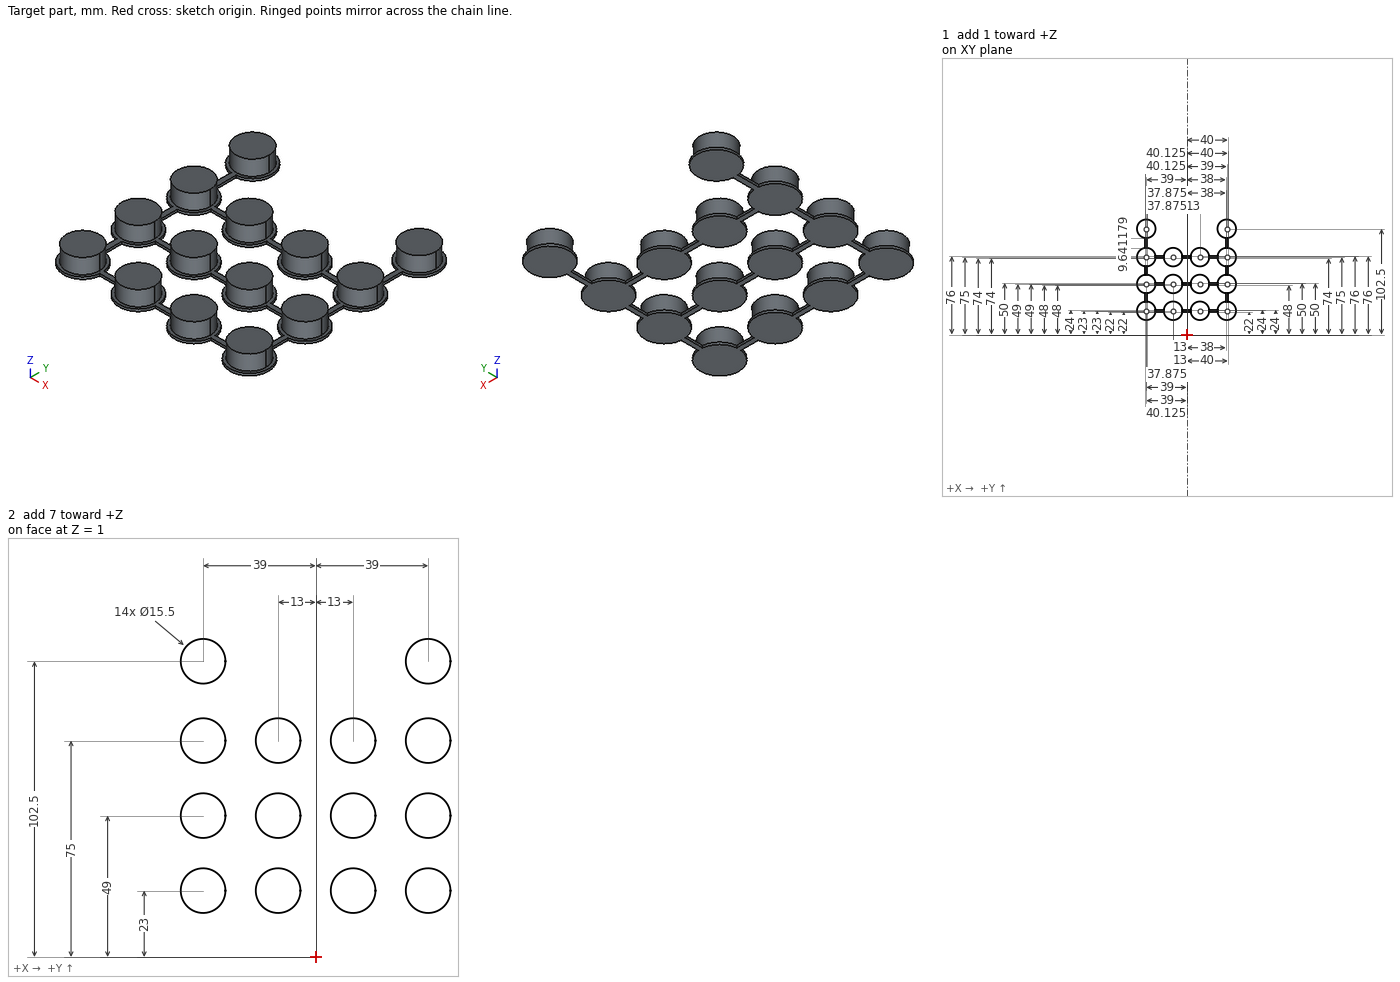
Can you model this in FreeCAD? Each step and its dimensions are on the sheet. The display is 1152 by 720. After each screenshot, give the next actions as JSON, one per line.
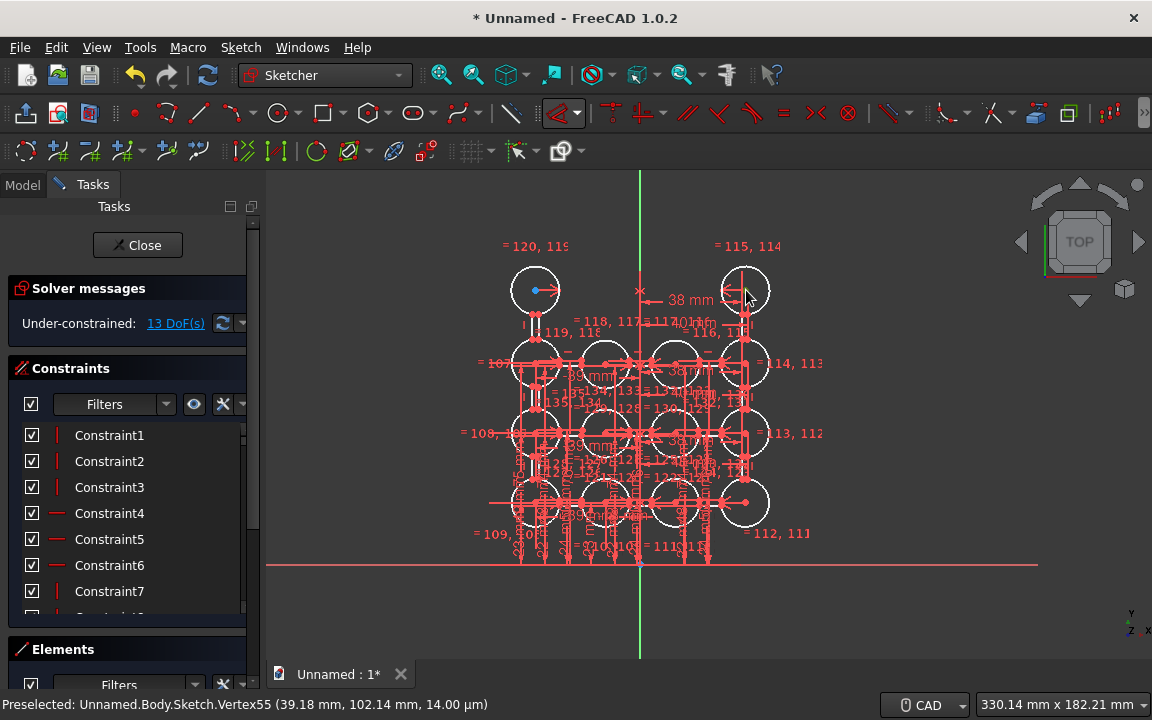
{"action": "key", "text": "l"}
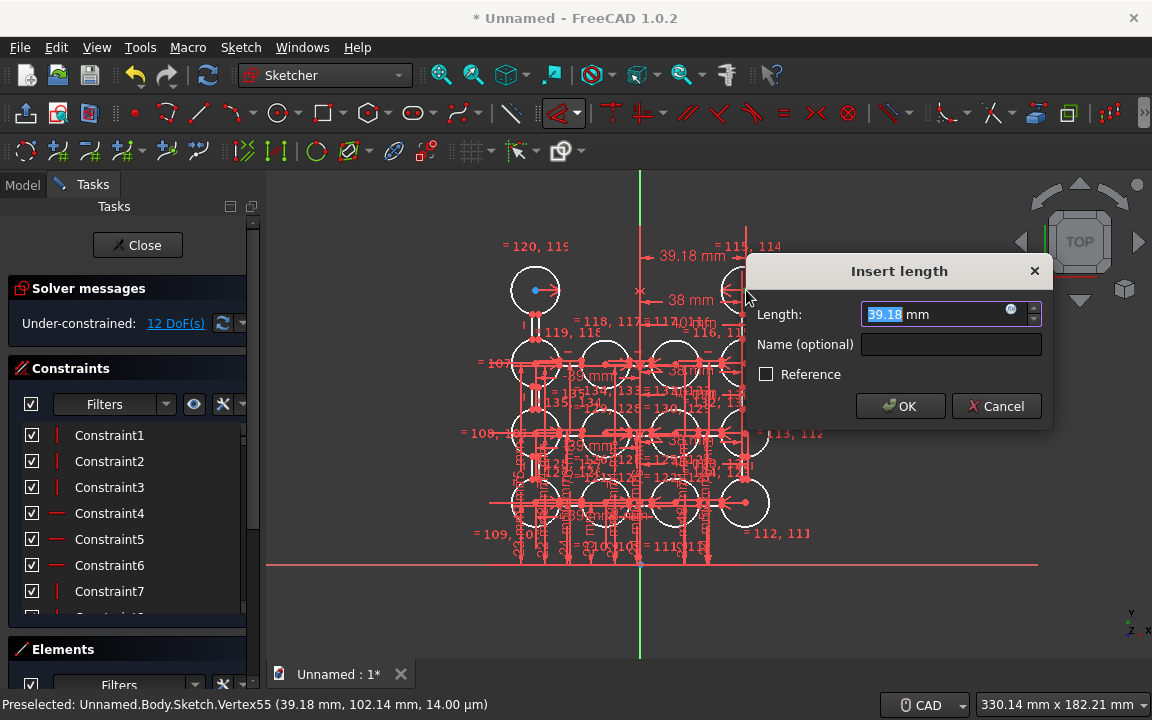
{"action": "type", "text": "39"}
{"action": "key", "text": "Return"}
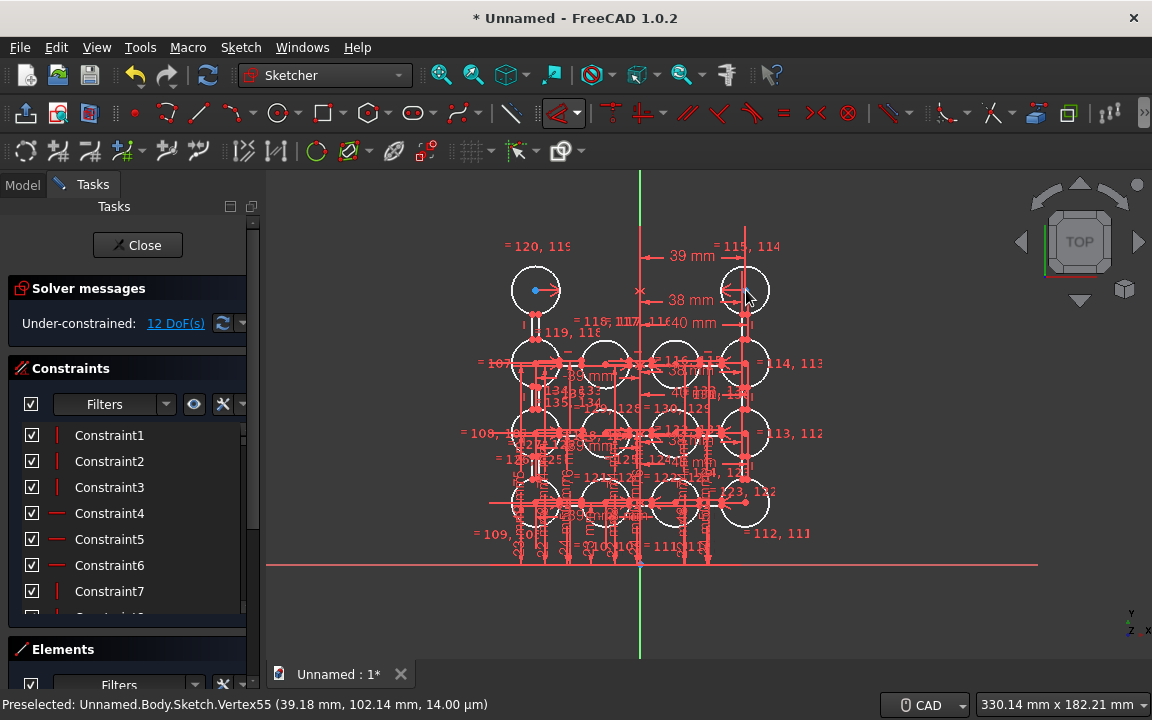
{"action": "left_click", "coordinate": [675, 365]}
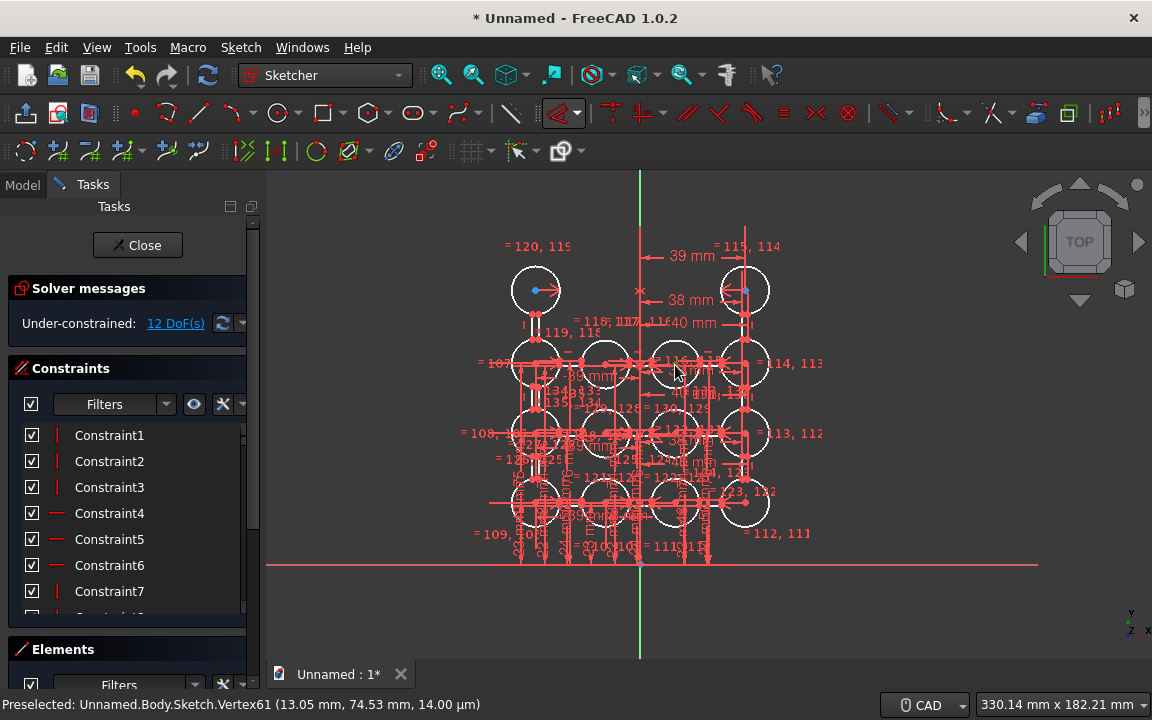
{"action": "left_click", "coordinate": [580, 114]}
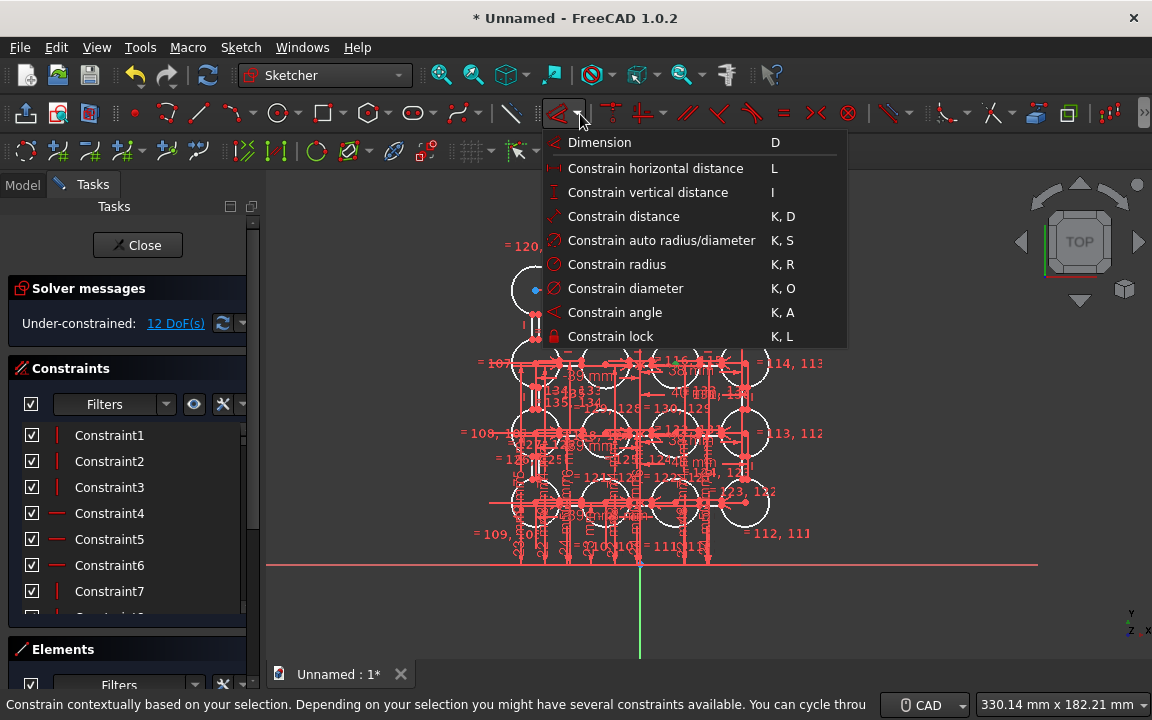
{"action": "left_click", "coordinate": [695, 168]}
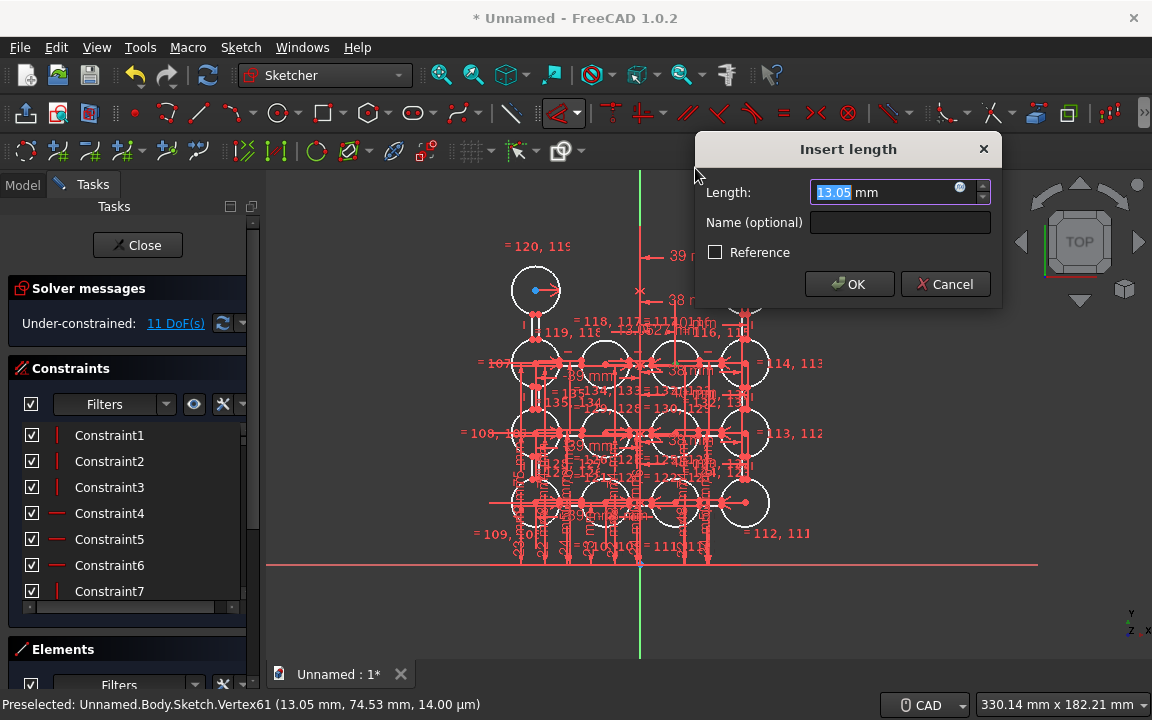
{"action": "type", "text": "13"}
{"action": "key", "text": "Return"}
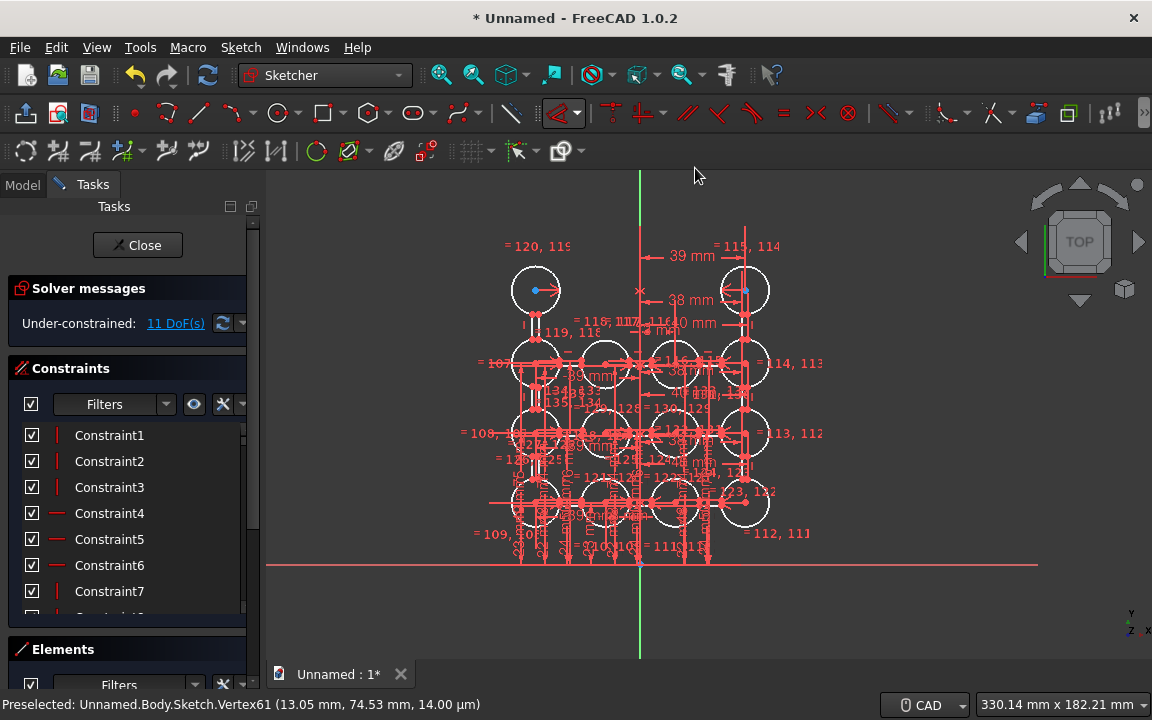
{"action": "left_click", "coordinate": [675, 365]}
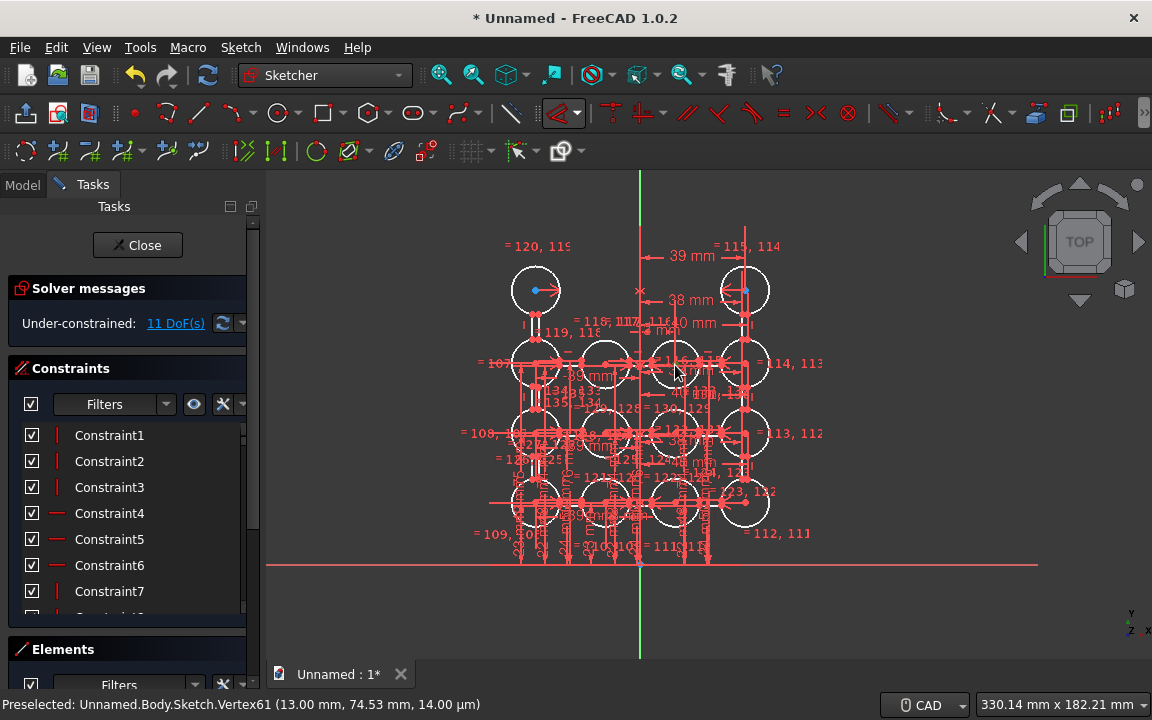
{"action": "key", "text": "i"}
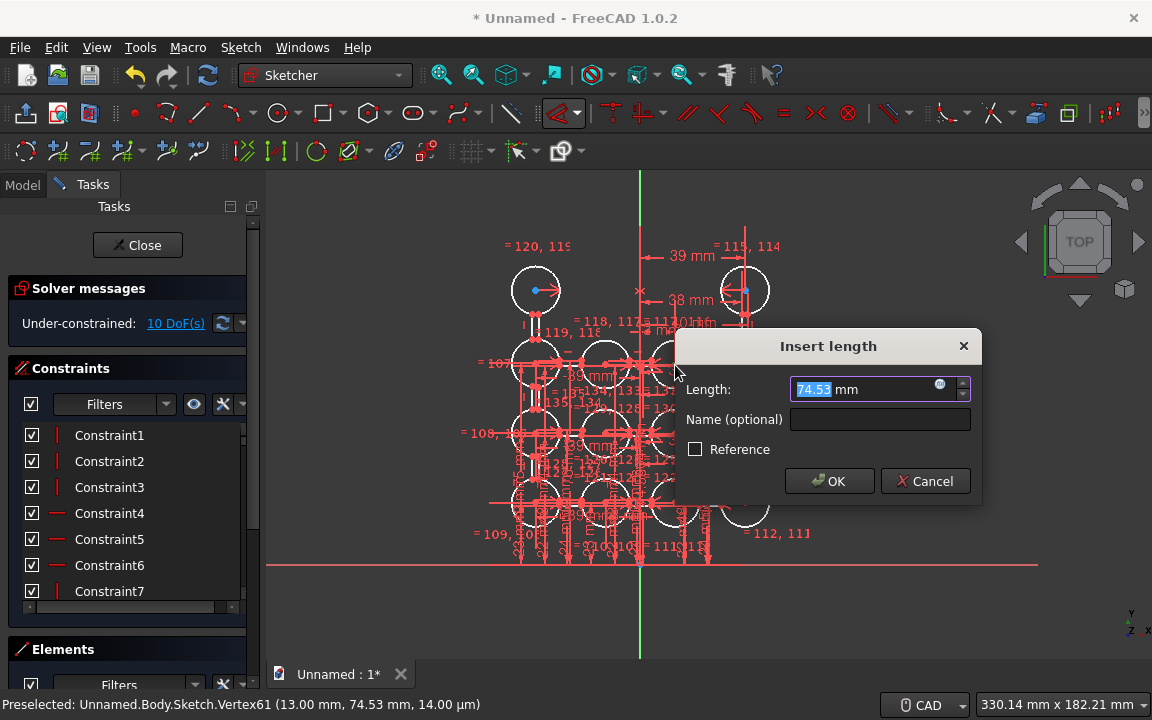
{"action": "type", "text": "75"}
{"action": "key", "text": "Return"}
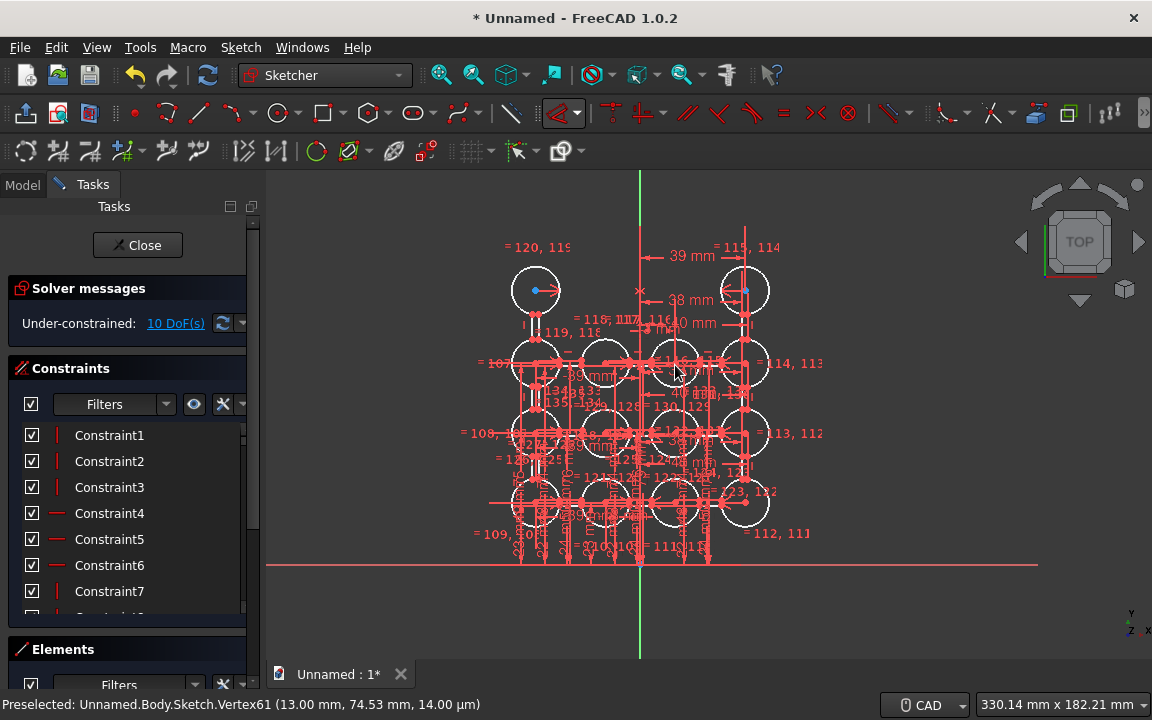
{"action": "left_click", "coordinate": [606, 434]}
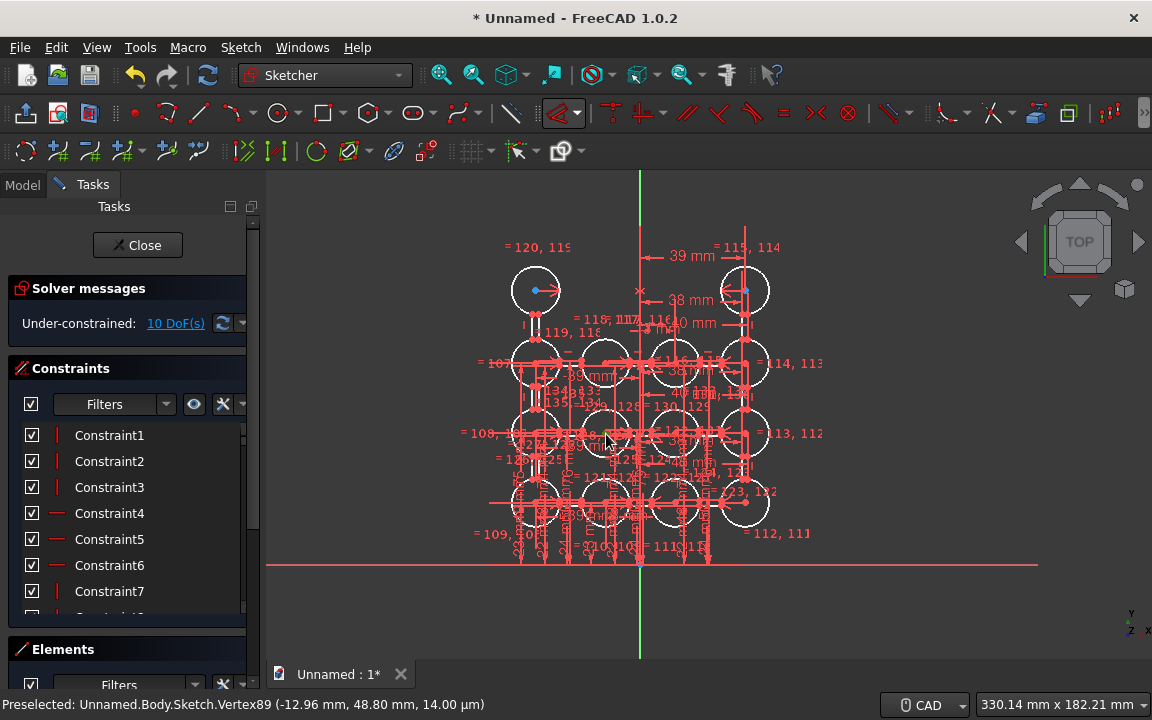
{"action": "left_click", "coordinate": [580, 114]}